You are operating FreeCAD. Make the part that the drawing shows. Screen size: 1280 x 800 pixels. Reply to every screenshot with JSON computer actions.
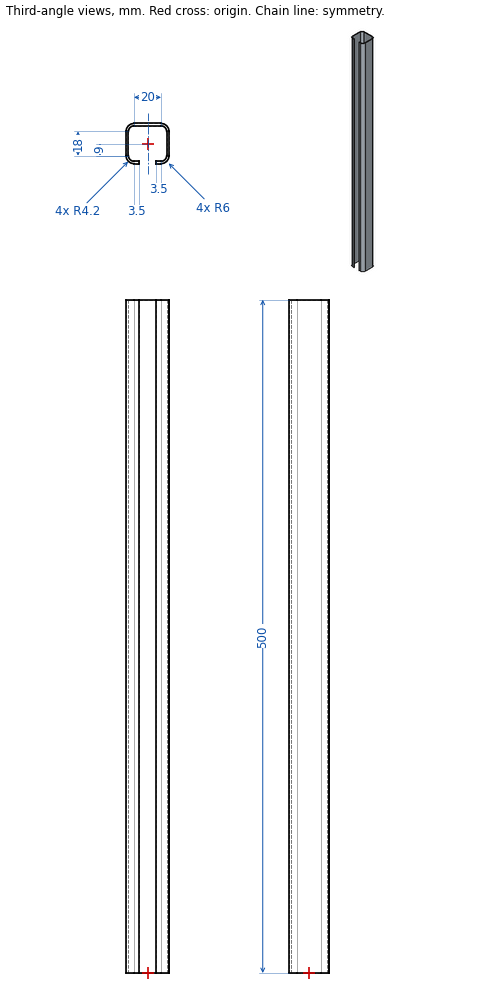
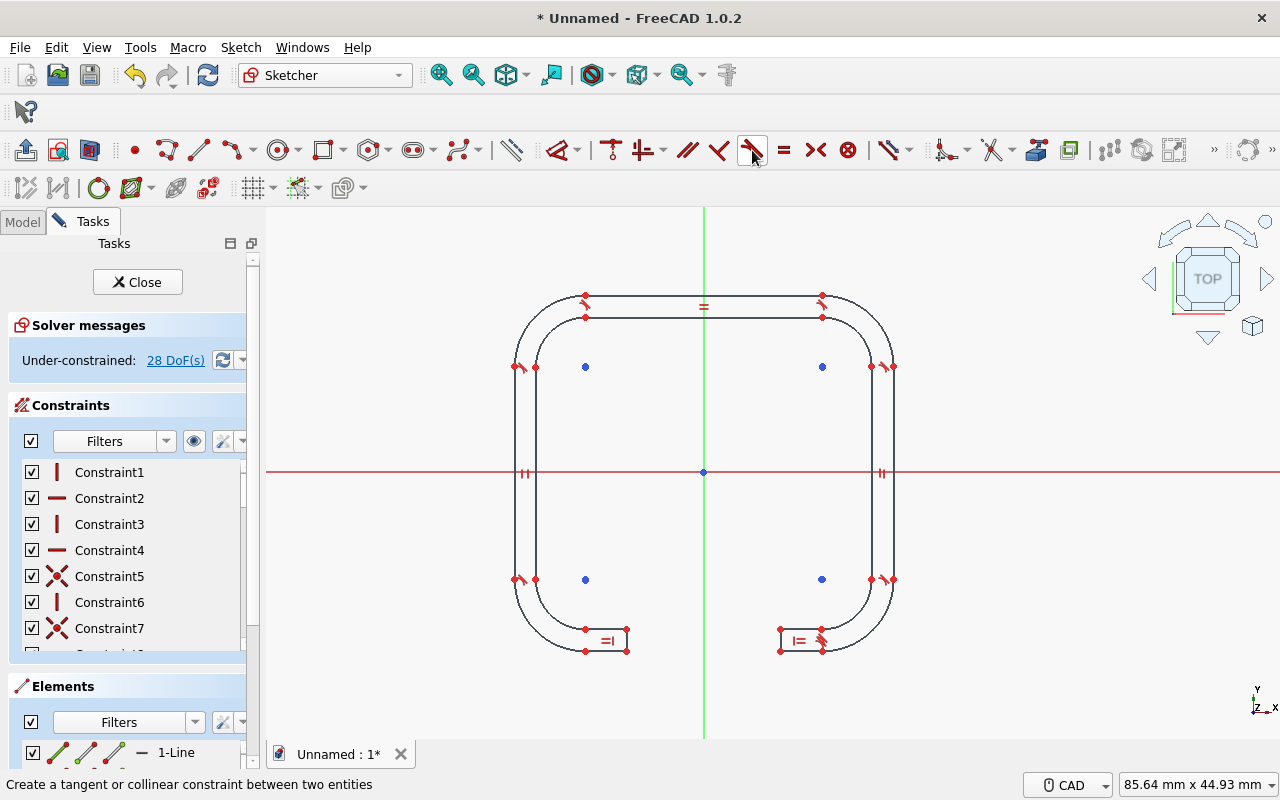
{"action": "left_click", "coordinate": [894, 516]}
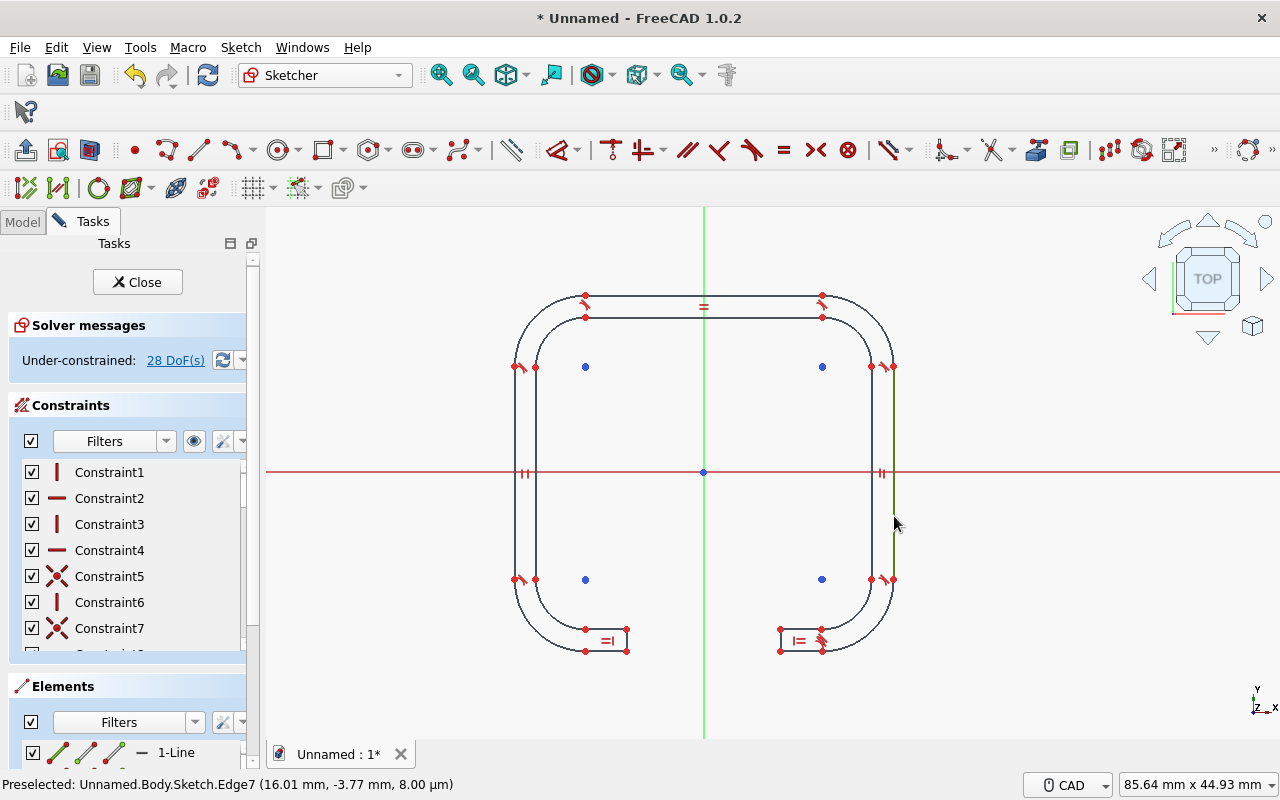
{"action": "left_click", "coordinate": [855, 644]}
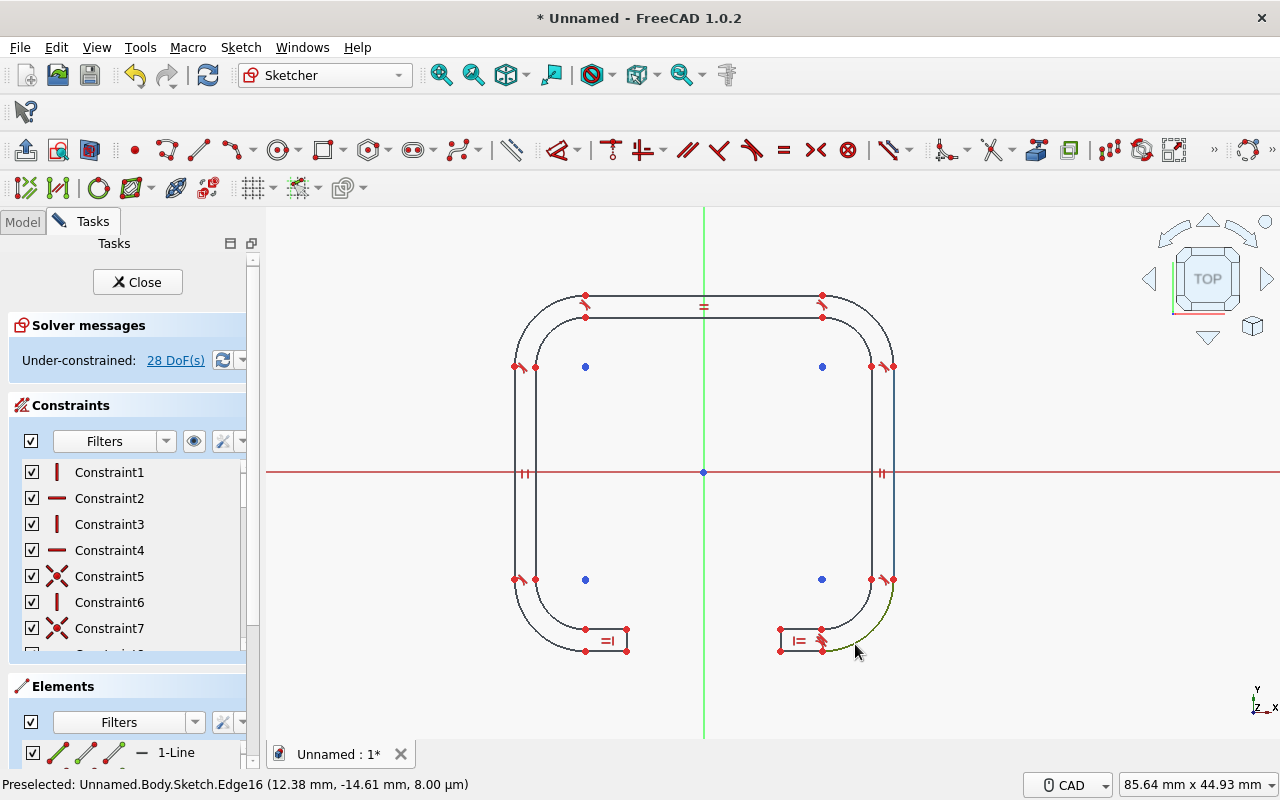
{"action": "left_click", "coordinate": [752, 150]}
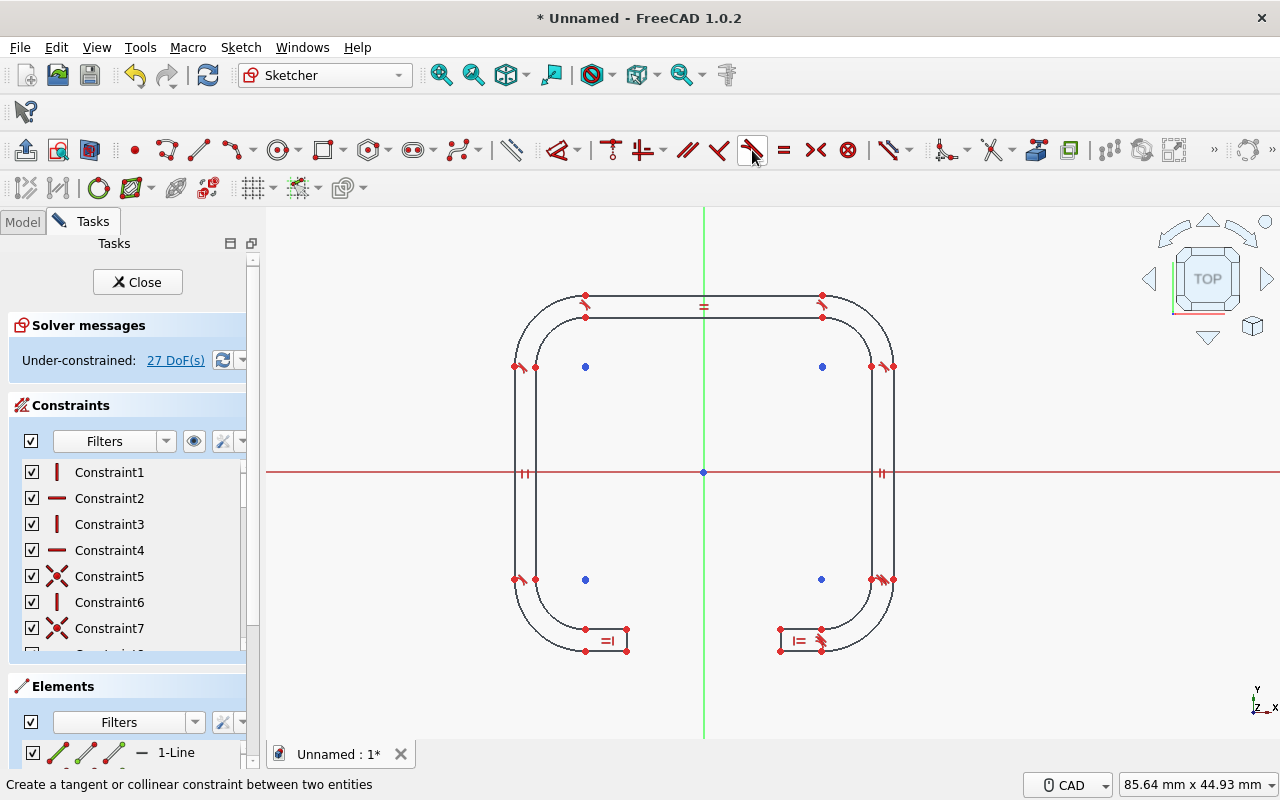
{"action": "left_click", "coordinate": [894, 516]}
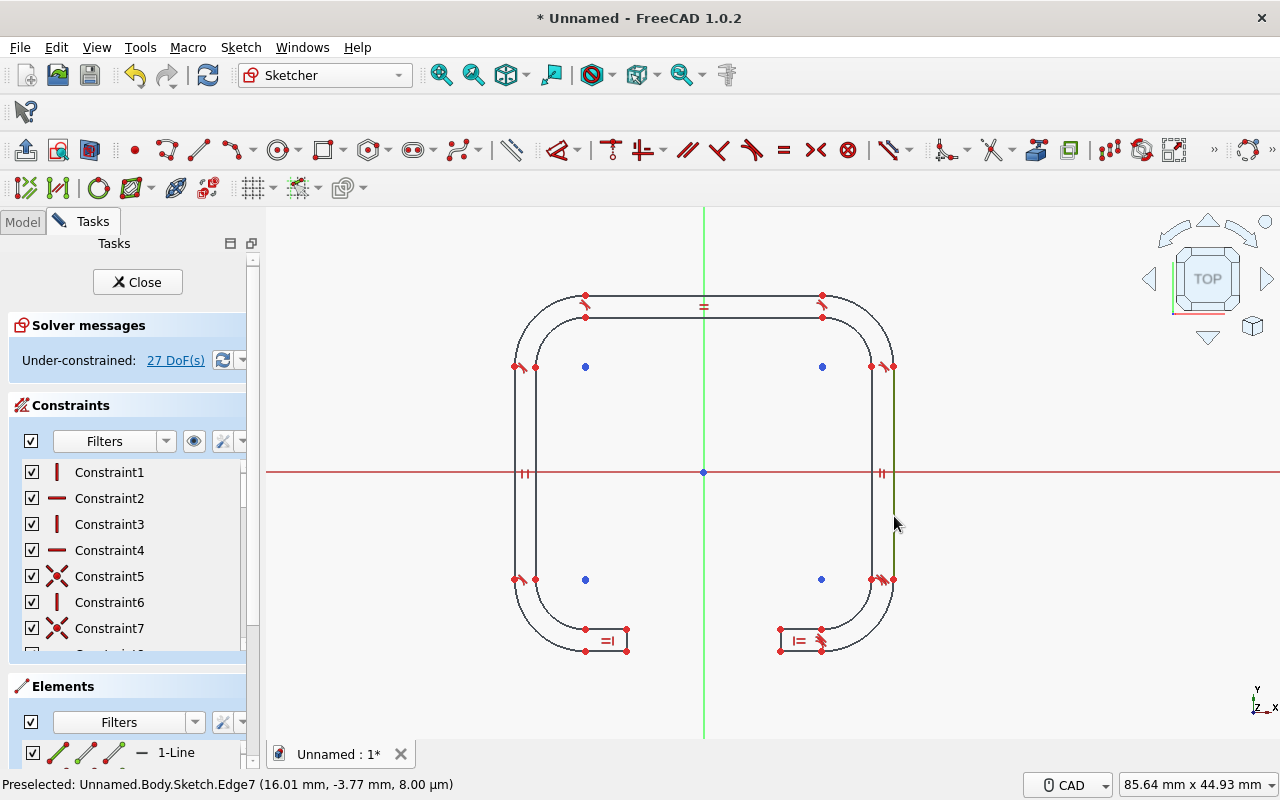
{"action": "left_click", "coordinate": [886, 334]}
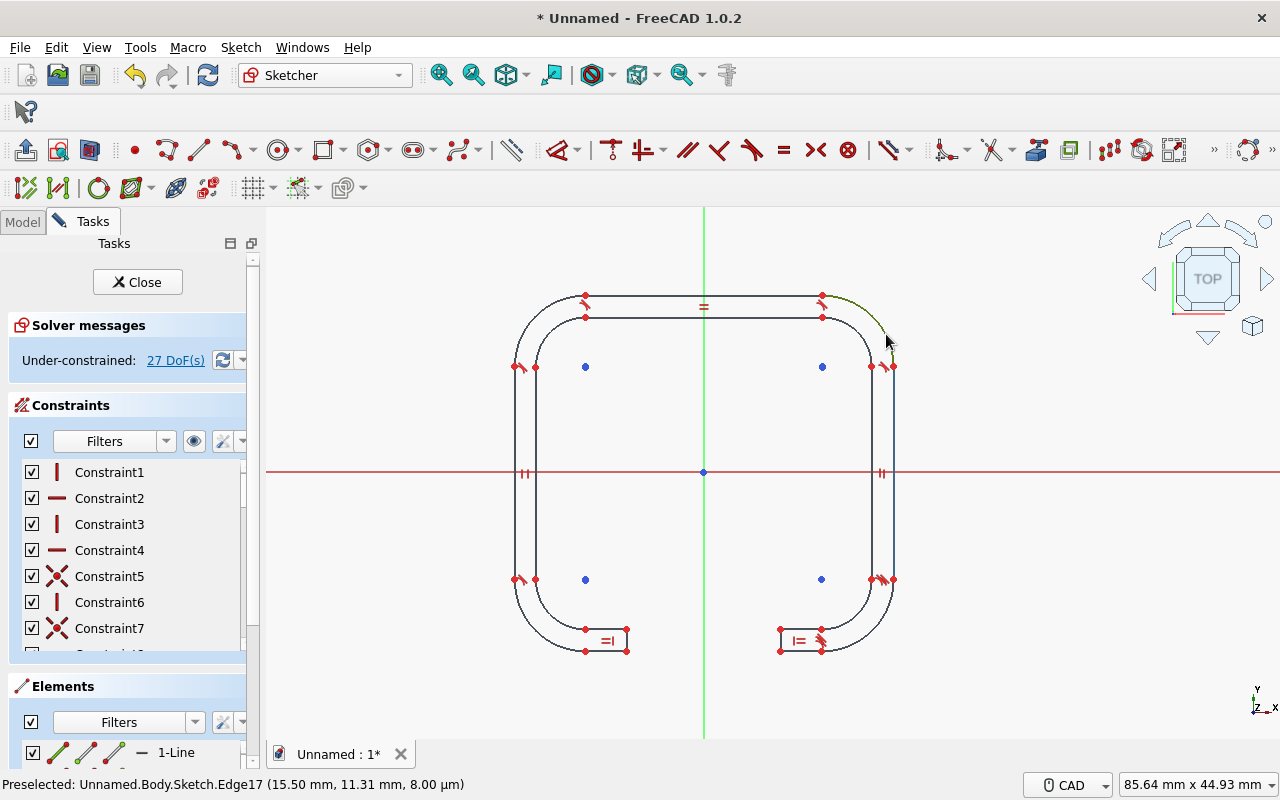
{"action": "left_click", "coordinate": [752, 150]}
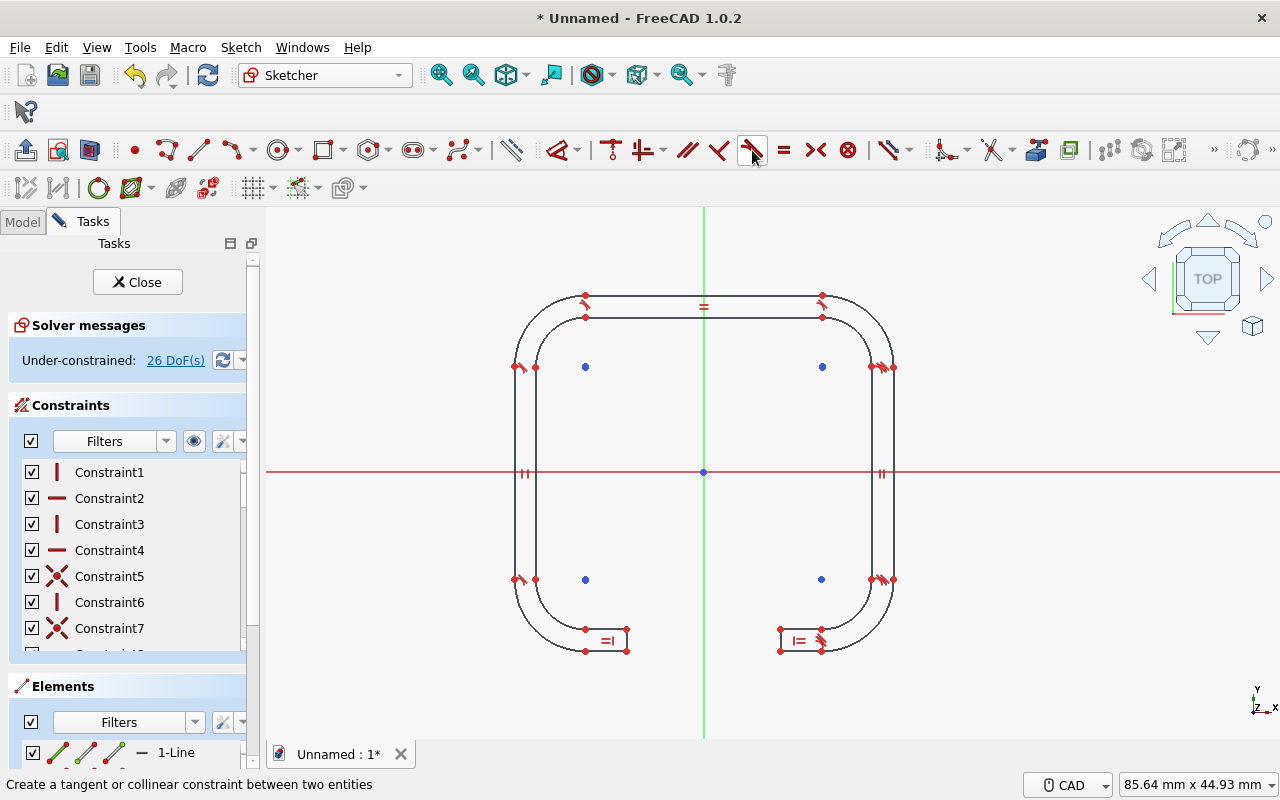
{"action": "left_click", "coordinate": [752, 296]}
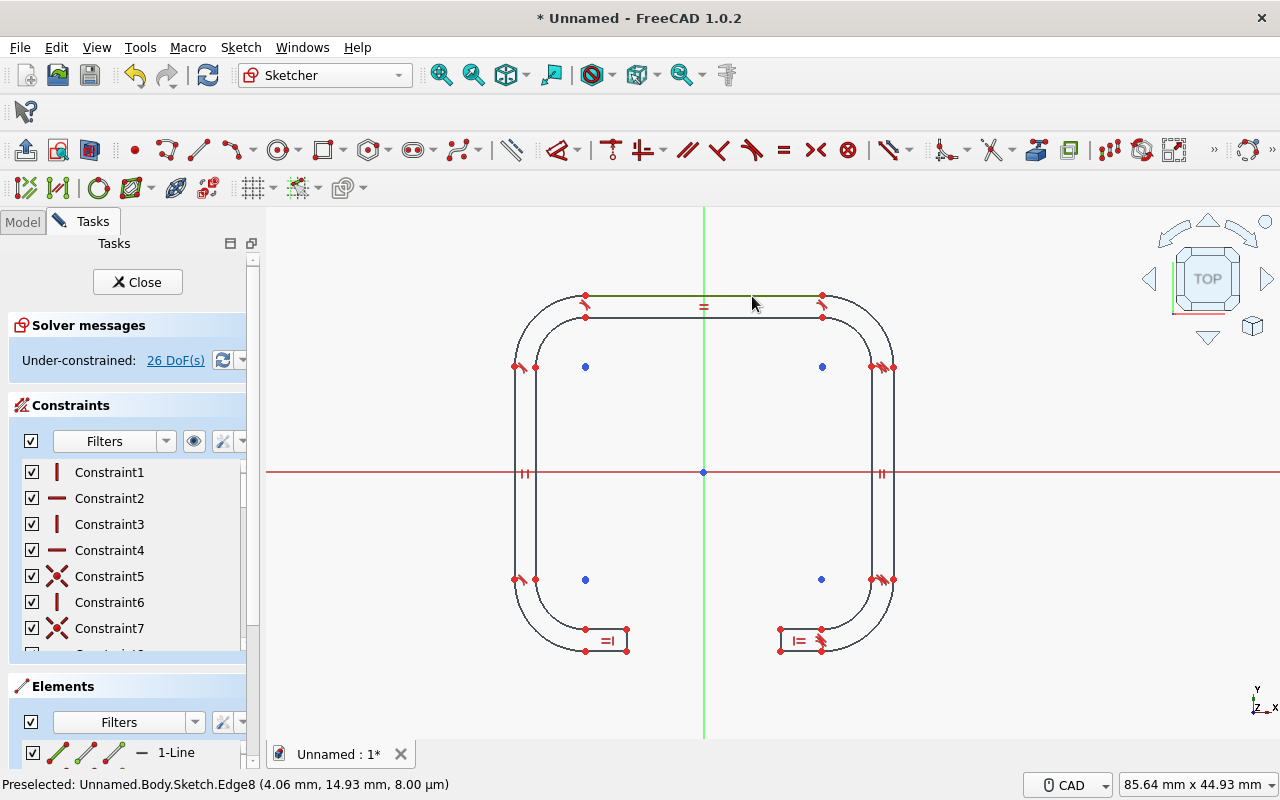
{"action": "left_click", "coordinate": [886, 335]}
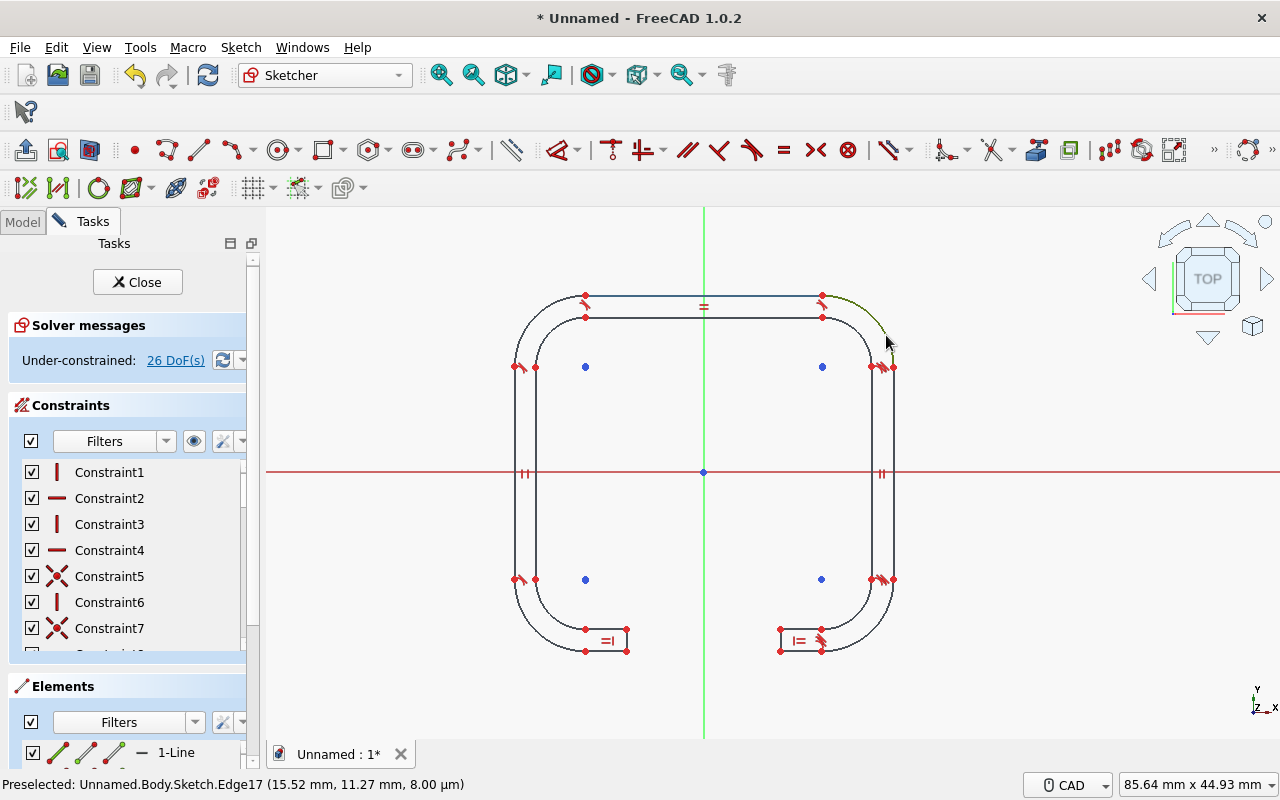
{"action": "left_click", "coordinate": [752, 150]}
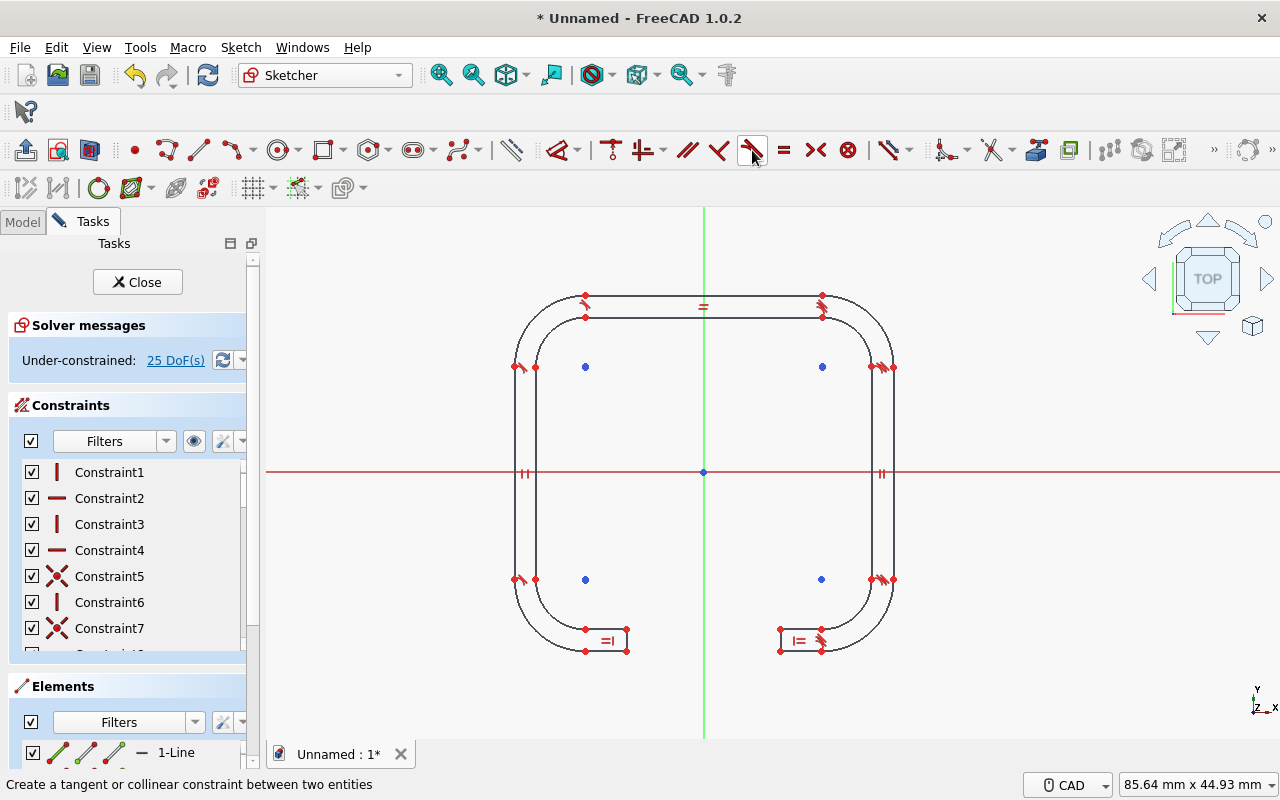
{"action": "left_click", "coordinate": [751, 296]}